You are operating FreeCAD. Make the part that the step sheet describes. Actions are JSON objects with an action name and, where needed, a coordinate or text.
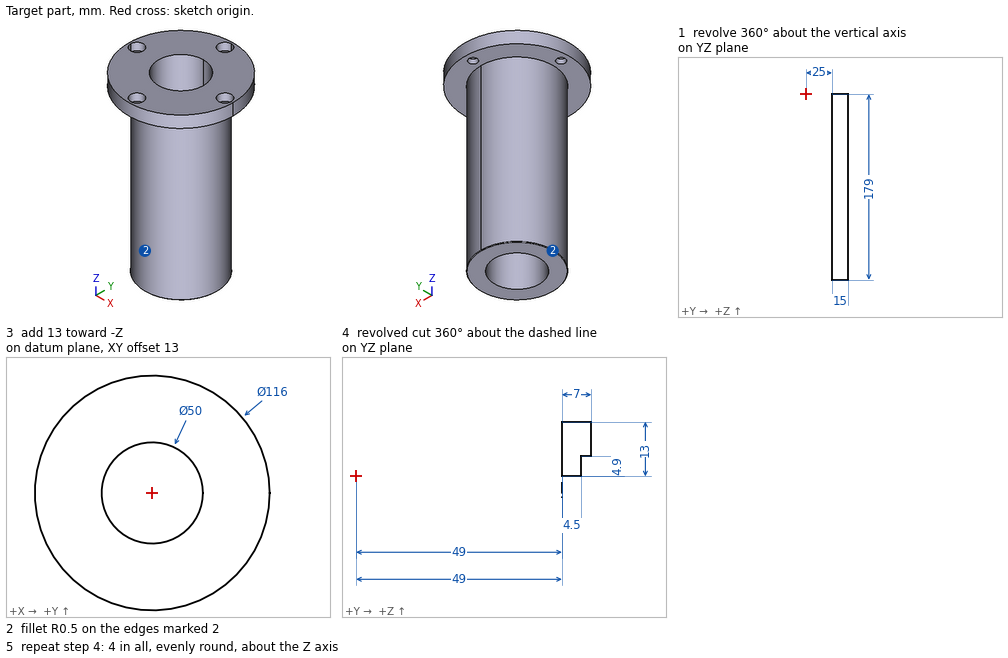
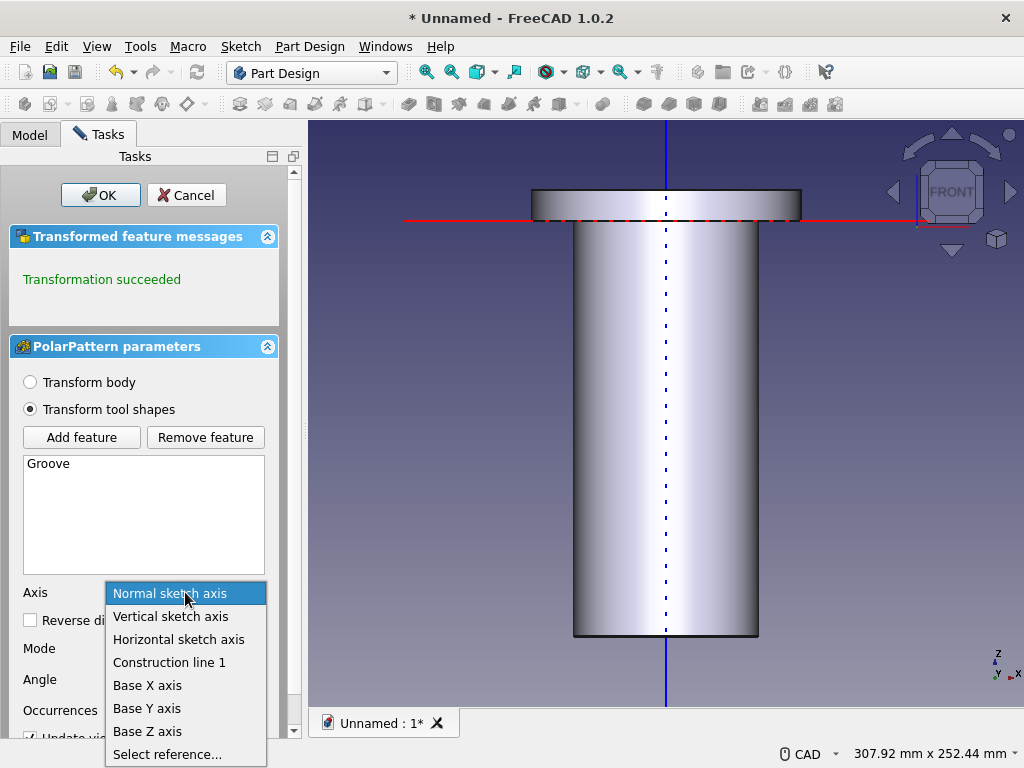
{"action": "left_click", "coordinate": [184, 732]}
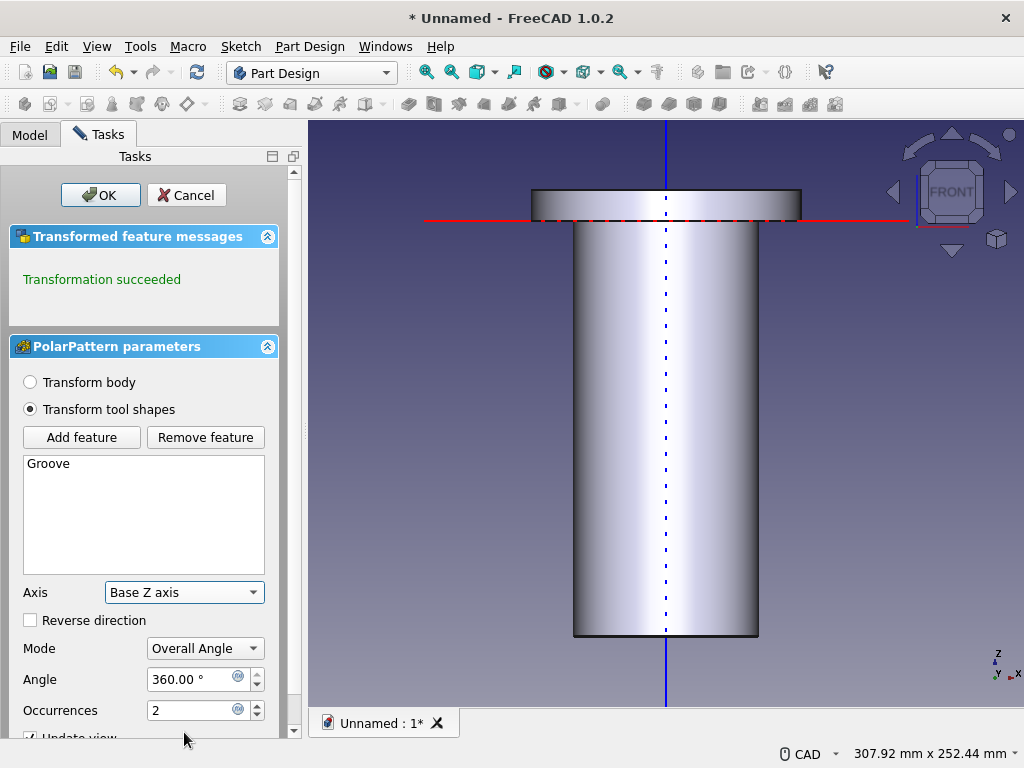
{"action": "triple_click", "coordinate": [199, 710]}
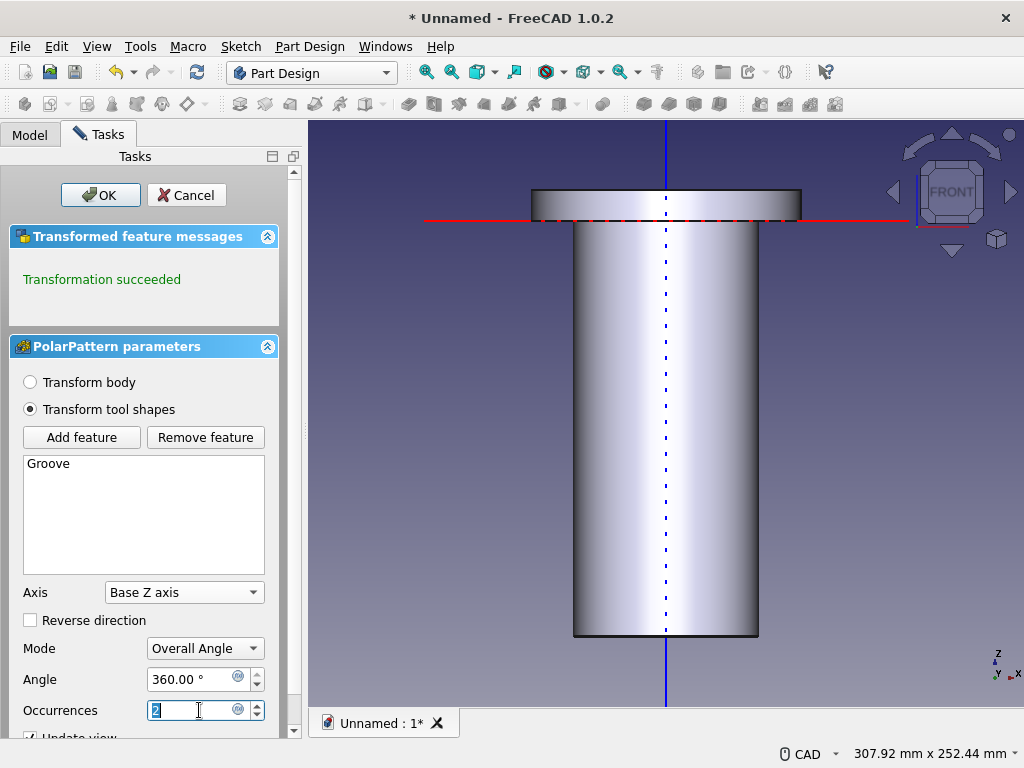
{"action": "type", "text": "4"}
{"action": "key", "text": "Tab"}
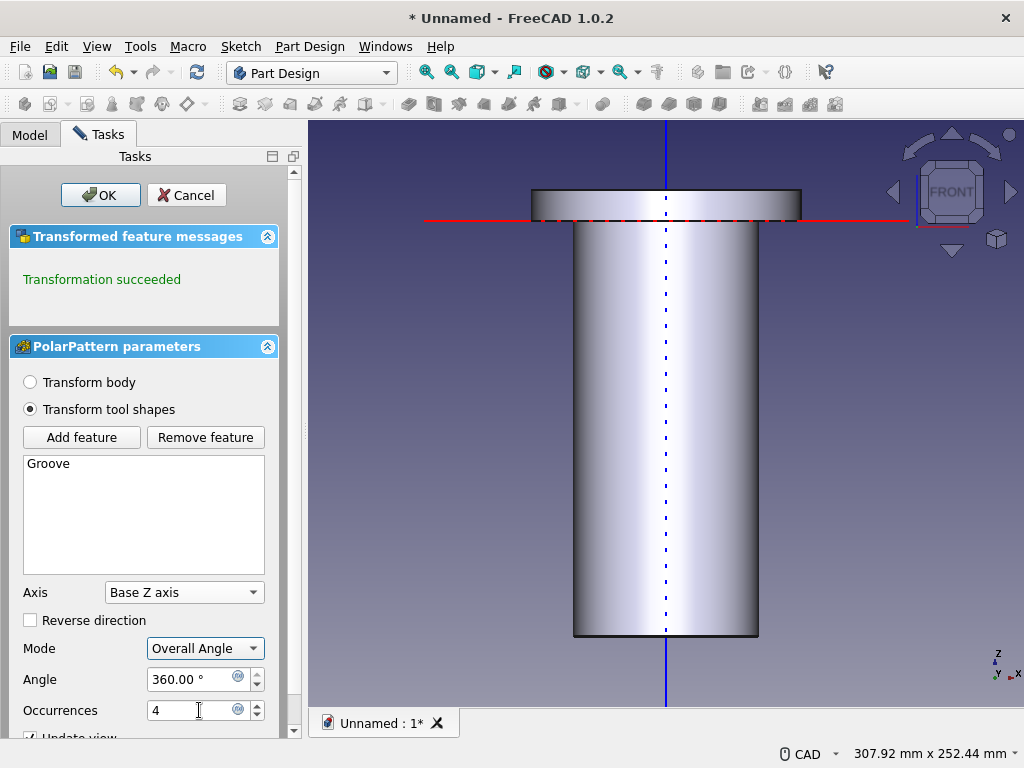
{"action": "left_click", "coordinate": [101, 195]}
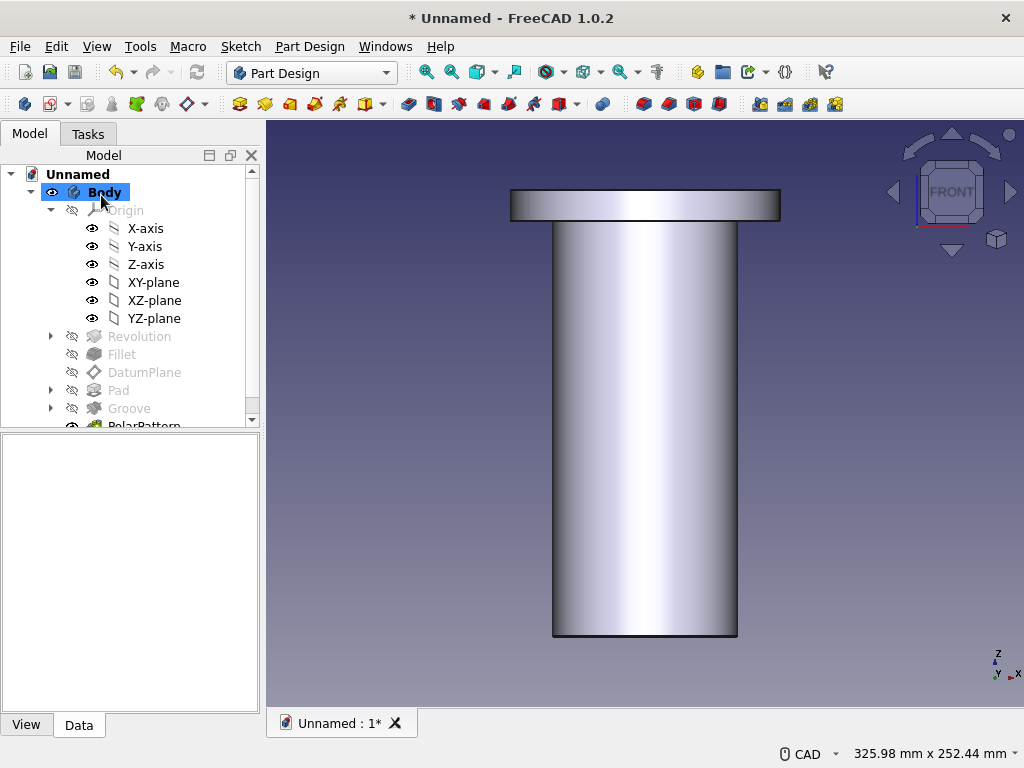
{"action": "key", "text": "0"}